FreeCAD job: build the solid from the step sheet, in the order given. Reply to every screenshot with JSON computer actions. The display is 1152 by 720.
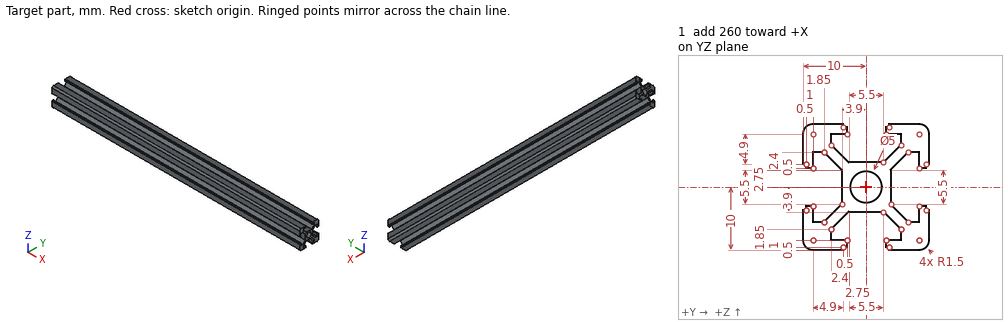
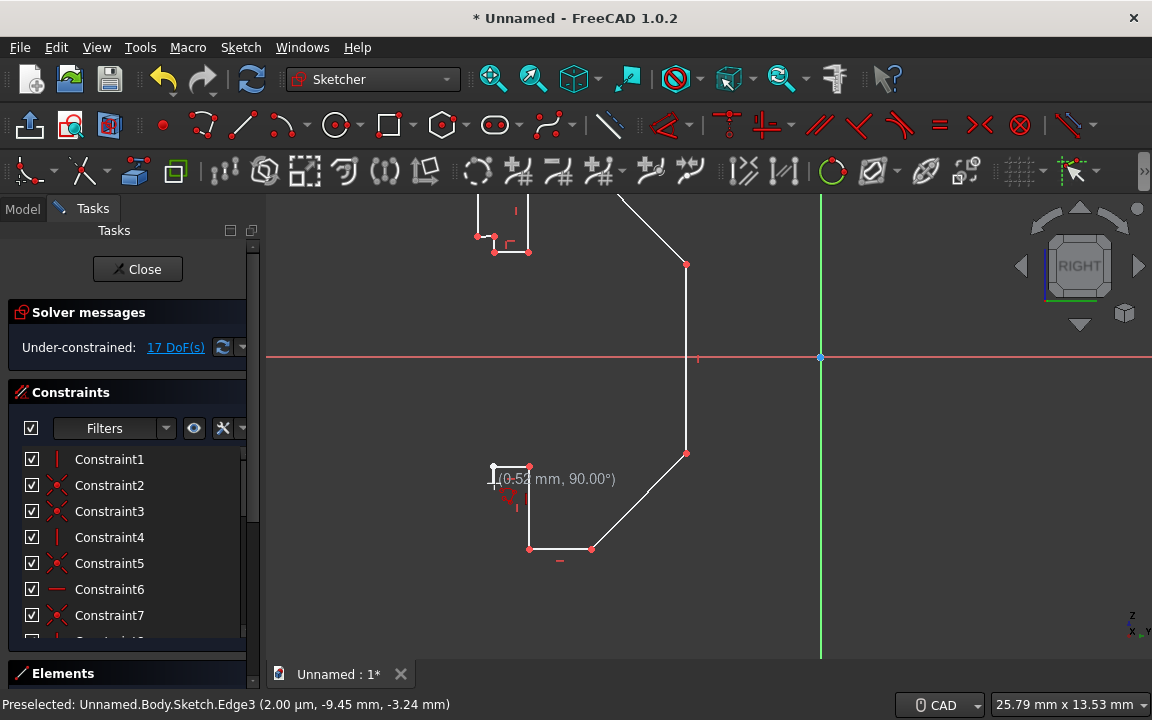
{"action": "left_click", "coordinate": [494, 481]}
{"action": "left_click", "coordinate": [477, 481]}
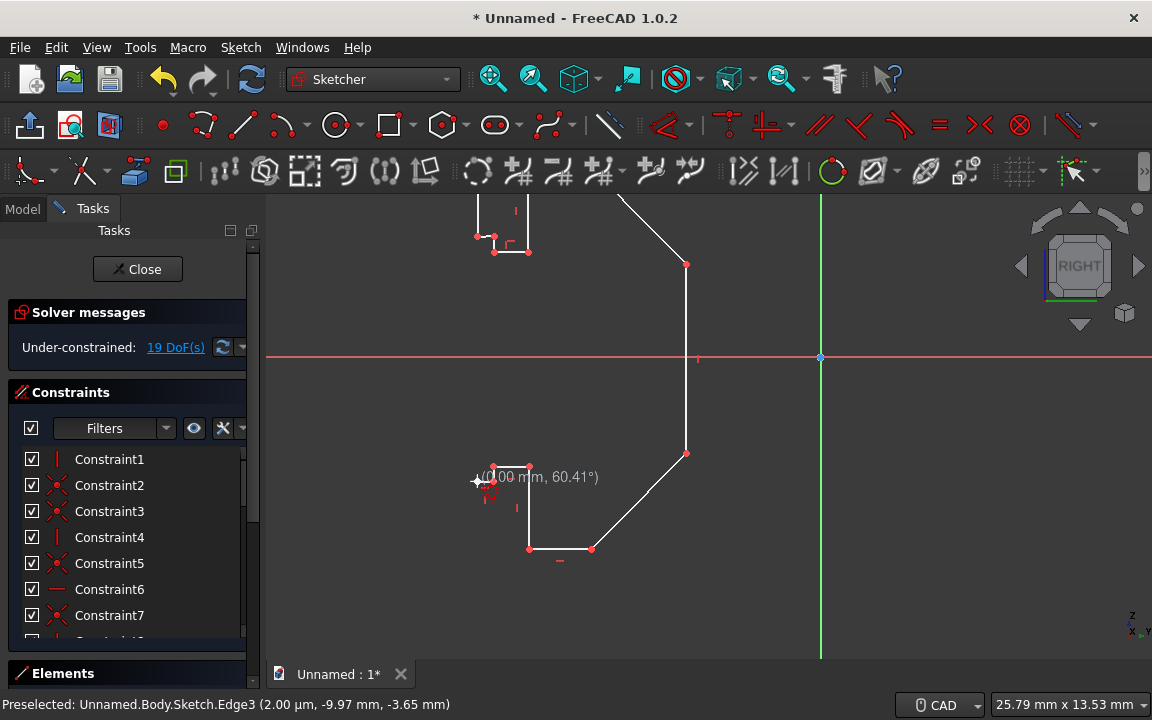
{"action": "scroll", "coordinate": [494, 483], "scroll_direction": "down", "scroll_amount": 4}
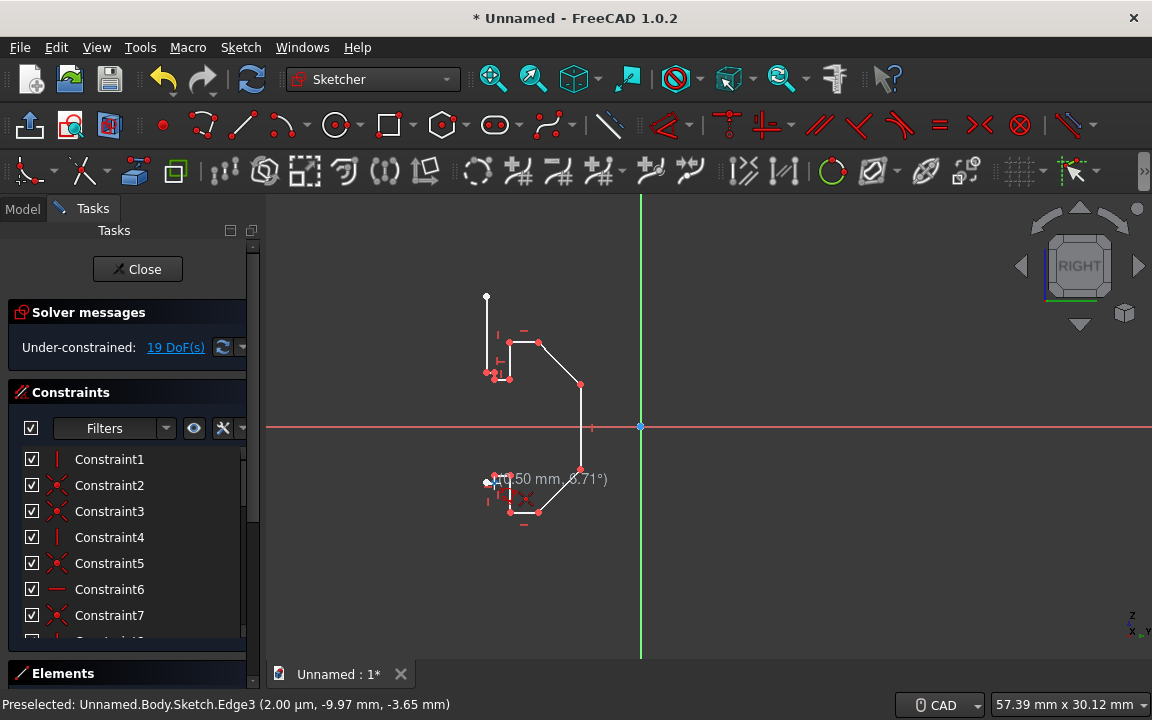
{"action": "left_click", "coordinate": [487, 558]}
{"action": "right_click", "coordinate": [487, 558]}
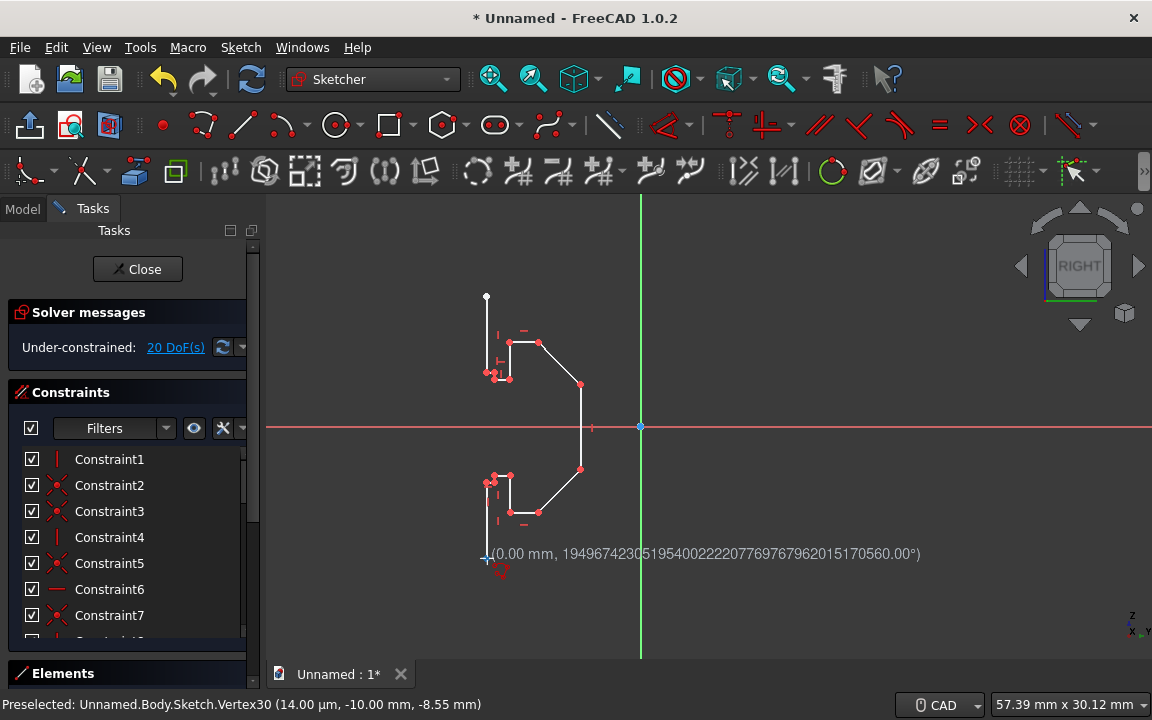
{"action": "left_click", "coordinate": [510, 581]}
{"action": "left_click", "coordinate": [585, 581]}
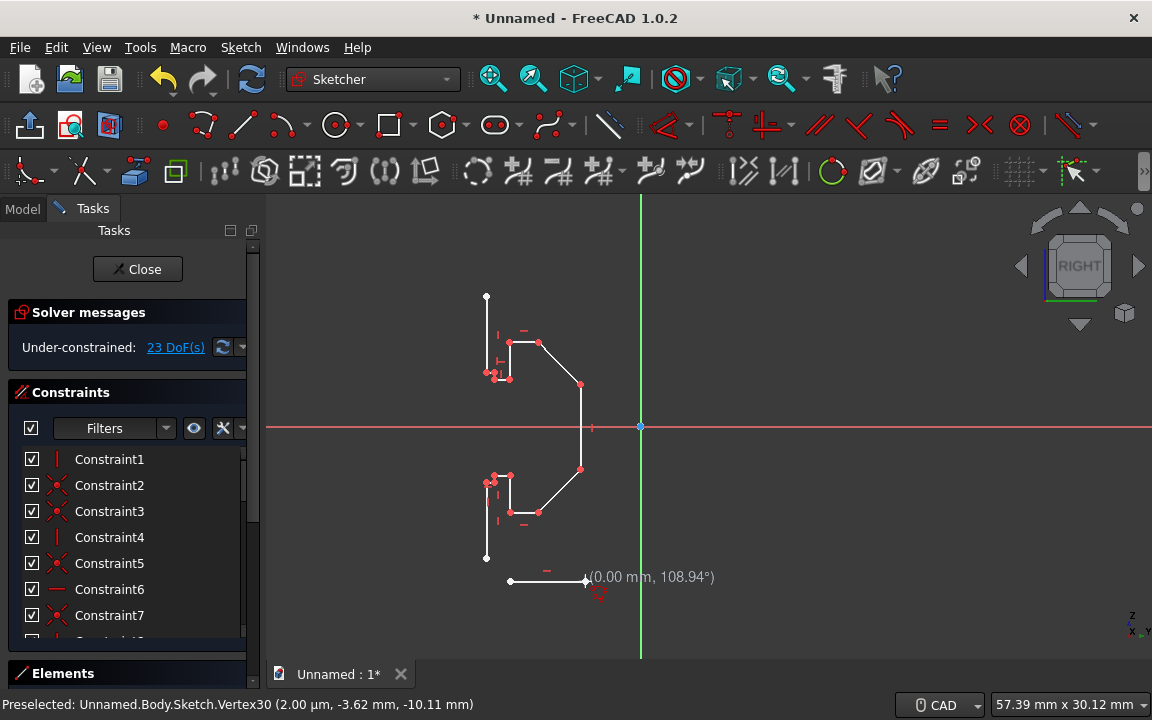
{"action": "scroll", "coordinate": [585, 574], "scroll_direction": "up", "scroll_amount": 4}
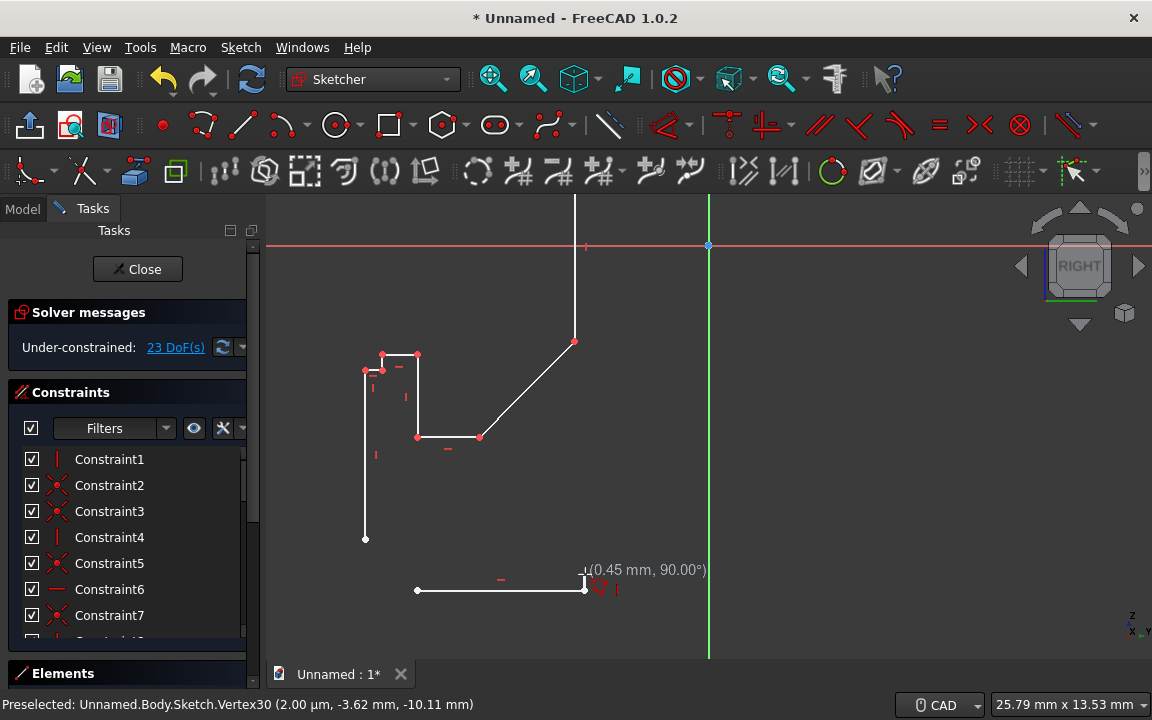
{"action": "left_click", "coordinate": [585, 572]}
{"action": "left_click", "coordinate": [602, 572]}
{"action": "left_click", "coordinate": [602, 538]}
{"action": "left_click", "coordinate": [520, 538]}
{"action": "left_click", "coordinate": [520, 474]}
{"action": "left_click", "coordinate": [615, 380]}
{"action": "left_click", "coordinate": [803, 380]}
{"action": "left_click", "coordinate": [898, 474]}
{"action": "left_click", "coordinate": [898, 538]}
{"action": "left_click", "coordinate": [816, 538]}
{"action": "left_click", "coordinate": [816, 572]}
{"action": "left_click", "coordinate": [833, 572]}
{"action": "left_click", "coordinate": [833, 589]}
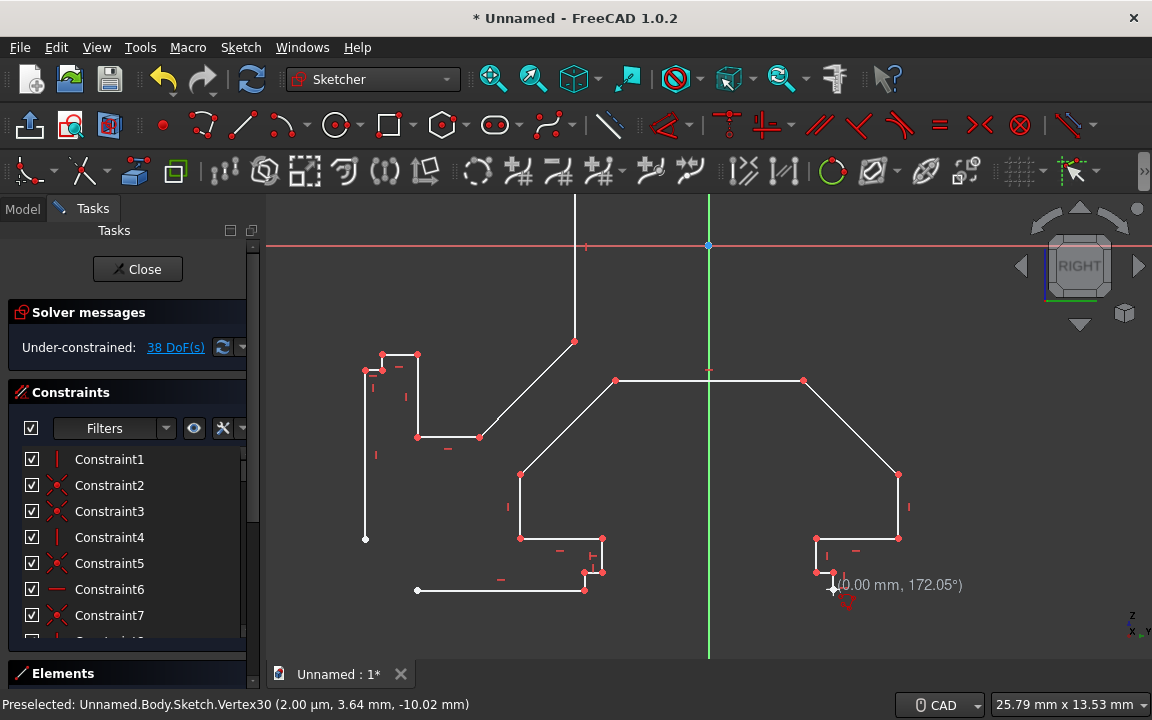
{"action": "scroll", "coordinate": [585, 574], "scroll_direction": "down", "scroll_amount": 4}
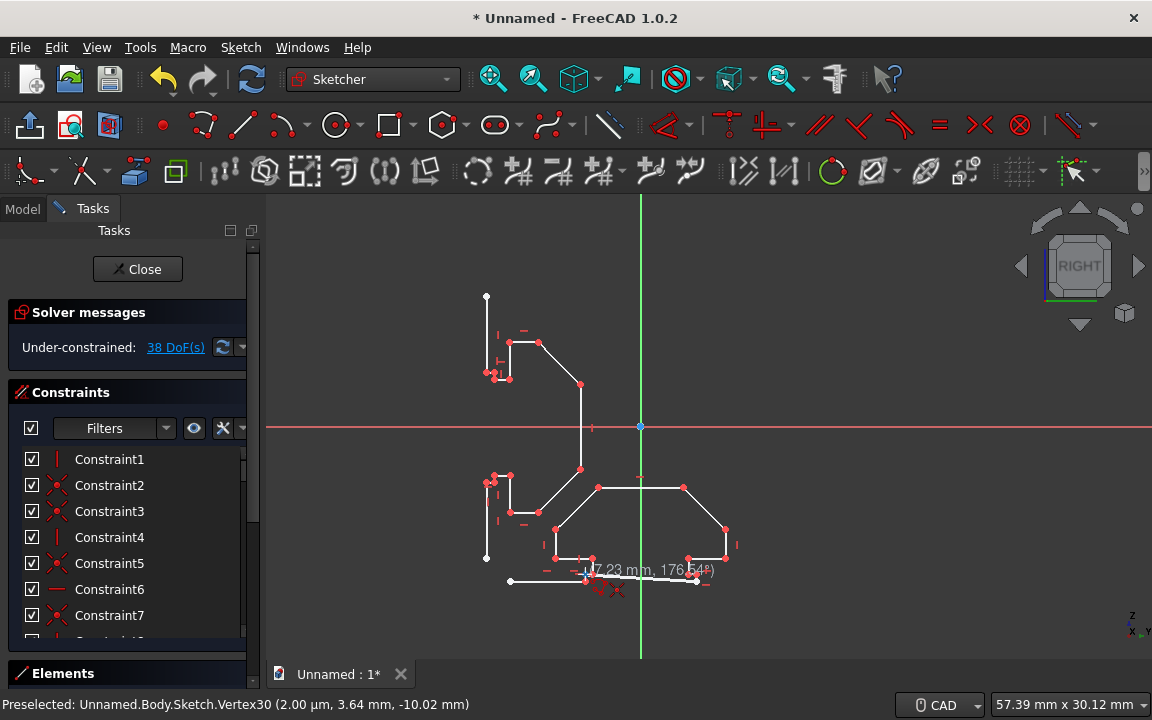
{"action": "left_click", "coordinate": [772, 581]}
{"action": "right_click", "coordinate": [772, 581]}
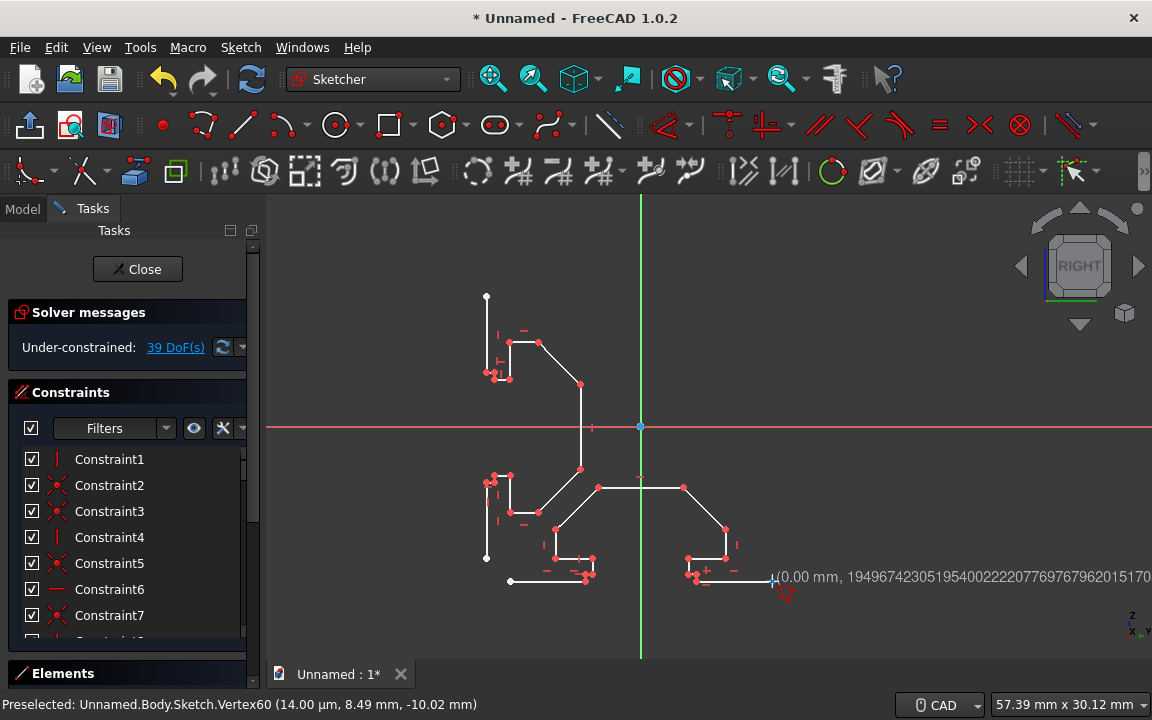
{"action": "left_click", "coordinate": [795, 558]}
{"action": "left_click", "coordinate": [795, 483]}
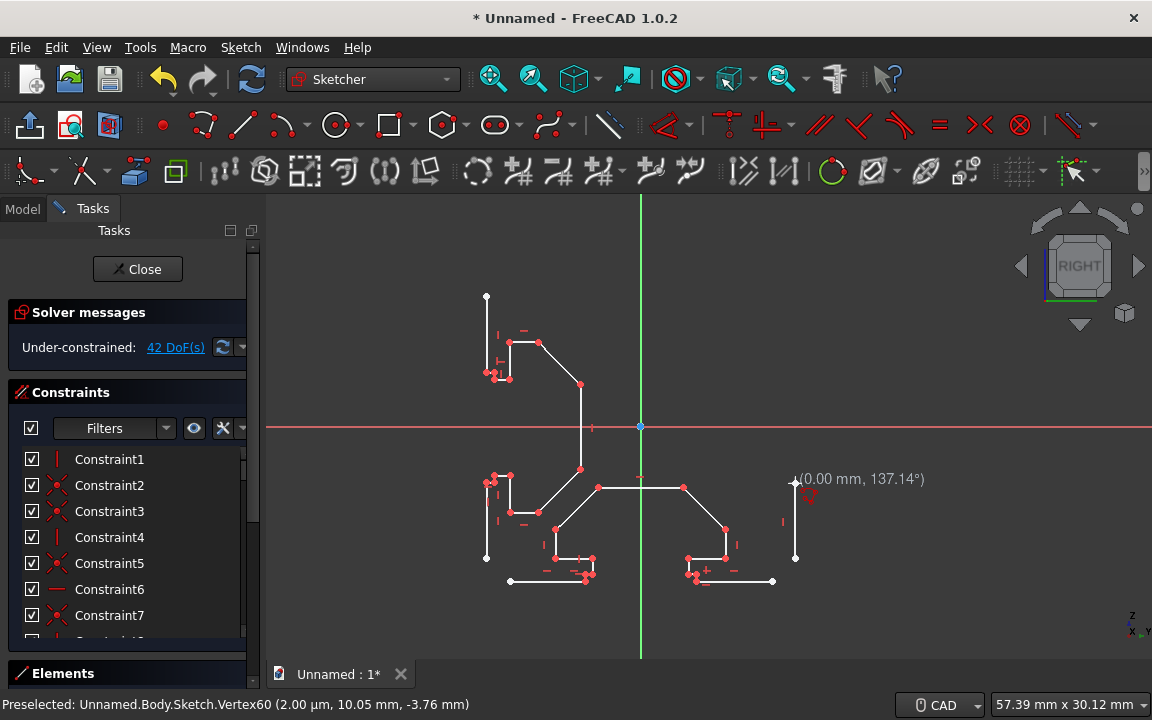
{"action": "scroll", "coordinate": [788, 483], "scroll_direction": "up", "scroll_amount": 4}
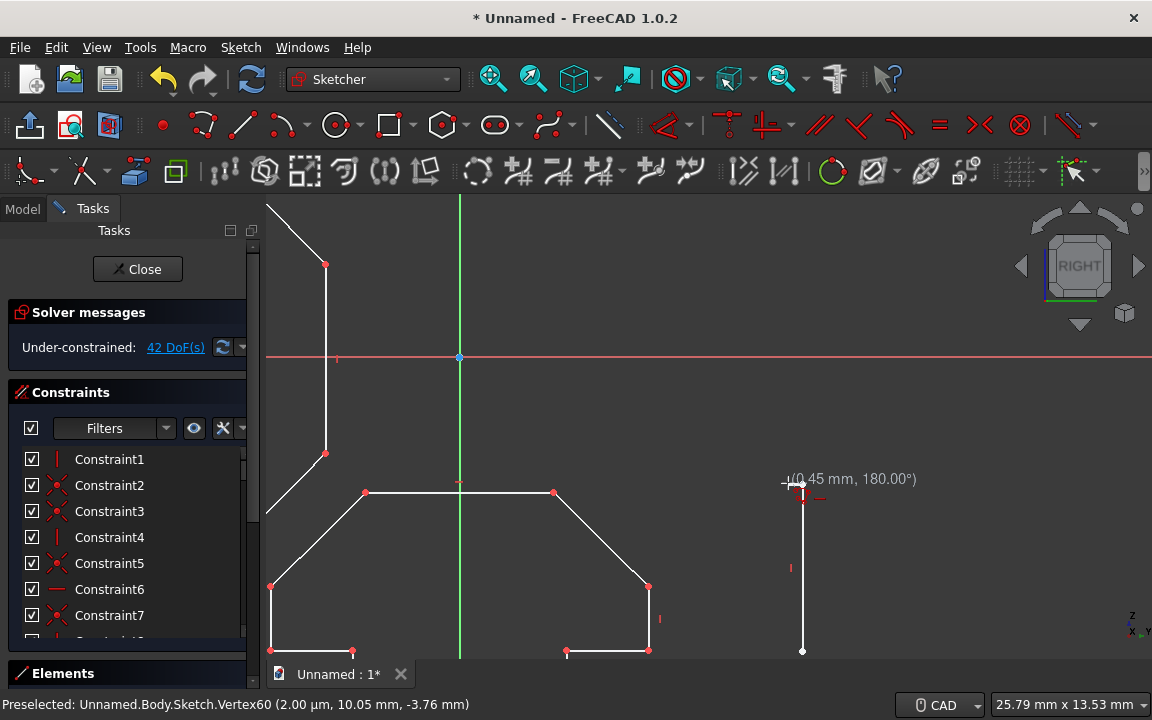
{"action": "left_click", "coordinate": [786, 482]}
{"action": "left_click", "coordinate": [786, 464]}
{"action": "left_click", "coordinate": [752, 464]}
{"action": "left_click", "coordinate": [752, 546]}
{"action": "left_click", "coordinate": [688, 546]}
{"action": "left_click", "coordinate": [594, 452]}
{"action": "left_click", "coordinate": [594, 263]}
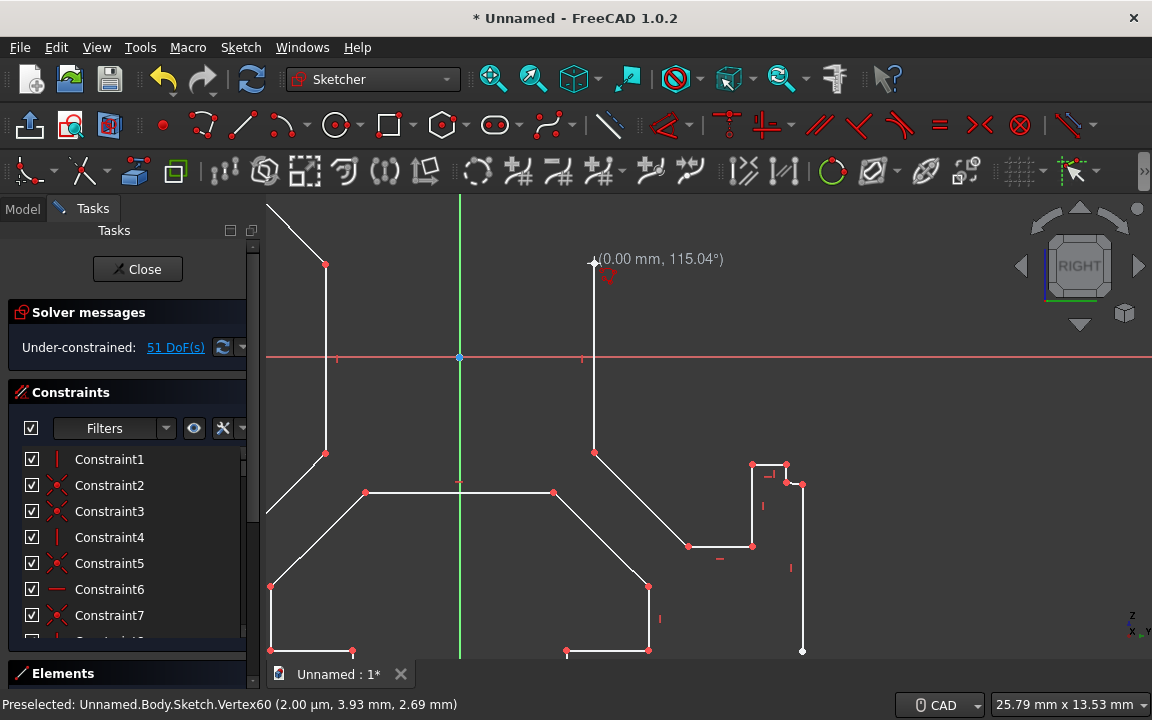
{"action": "scroll", "coordinate": [788, 483], "scroll_direction": "down", "scroll_amount": 4}